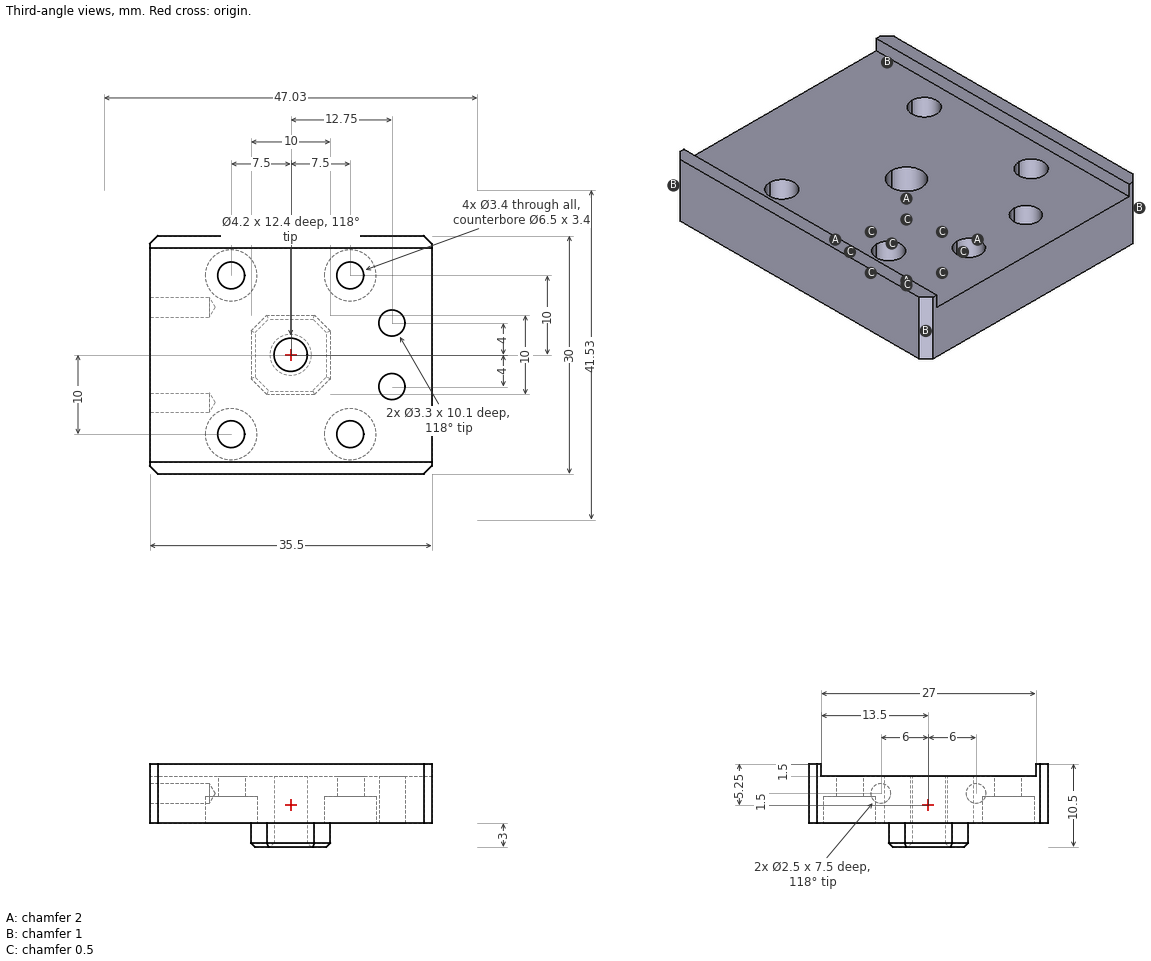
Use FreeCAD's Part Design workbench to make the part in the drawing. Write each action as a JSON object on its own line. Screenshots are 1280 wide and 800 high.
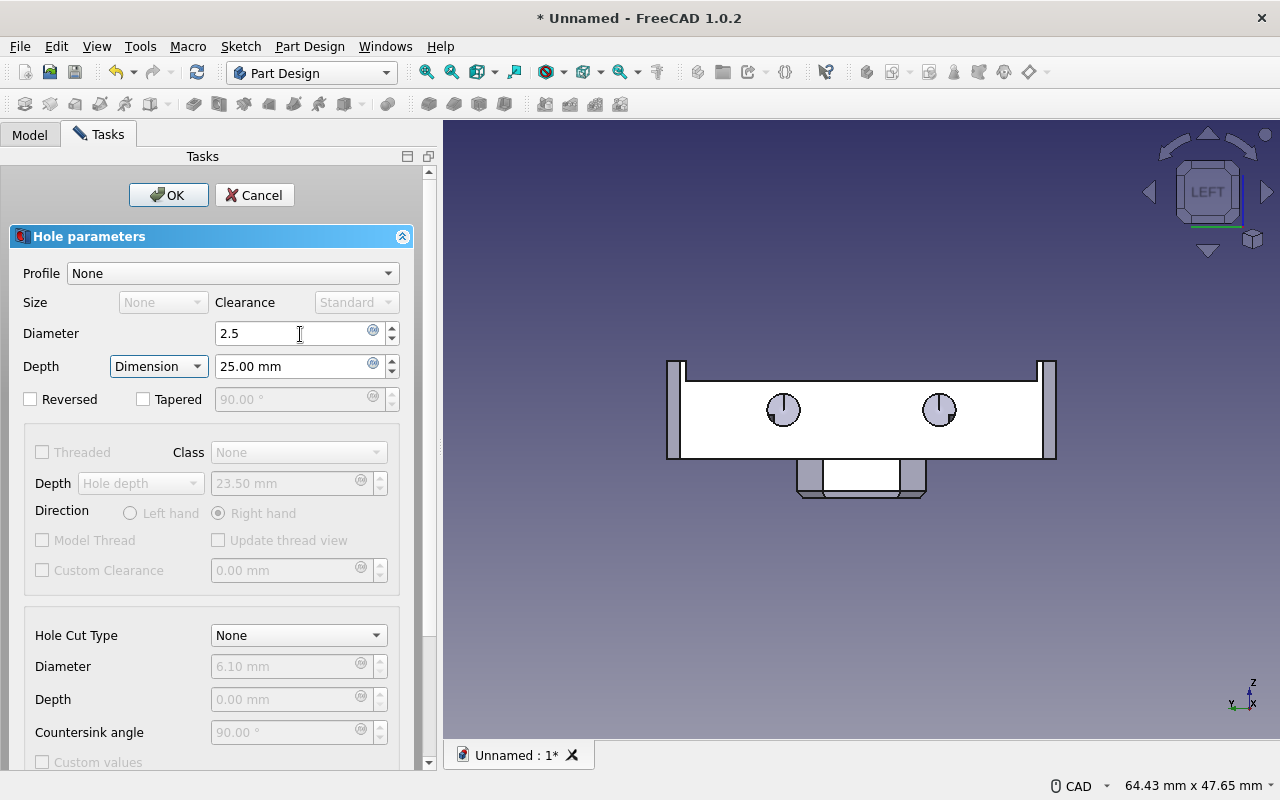
{"action": "triple_click", "coordinate": [300, 366]}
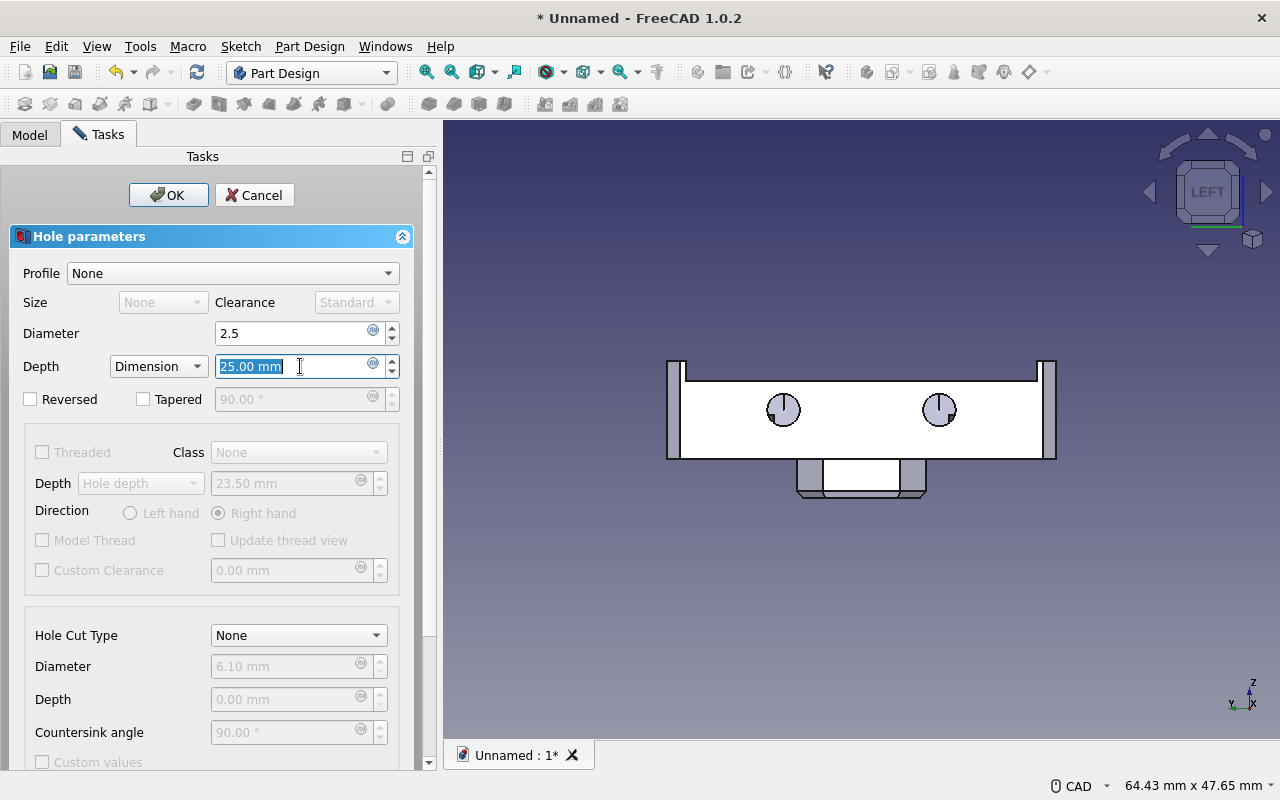
{"action": "type", "text": "7.5"}
{"action": "key", "text": "Tab"}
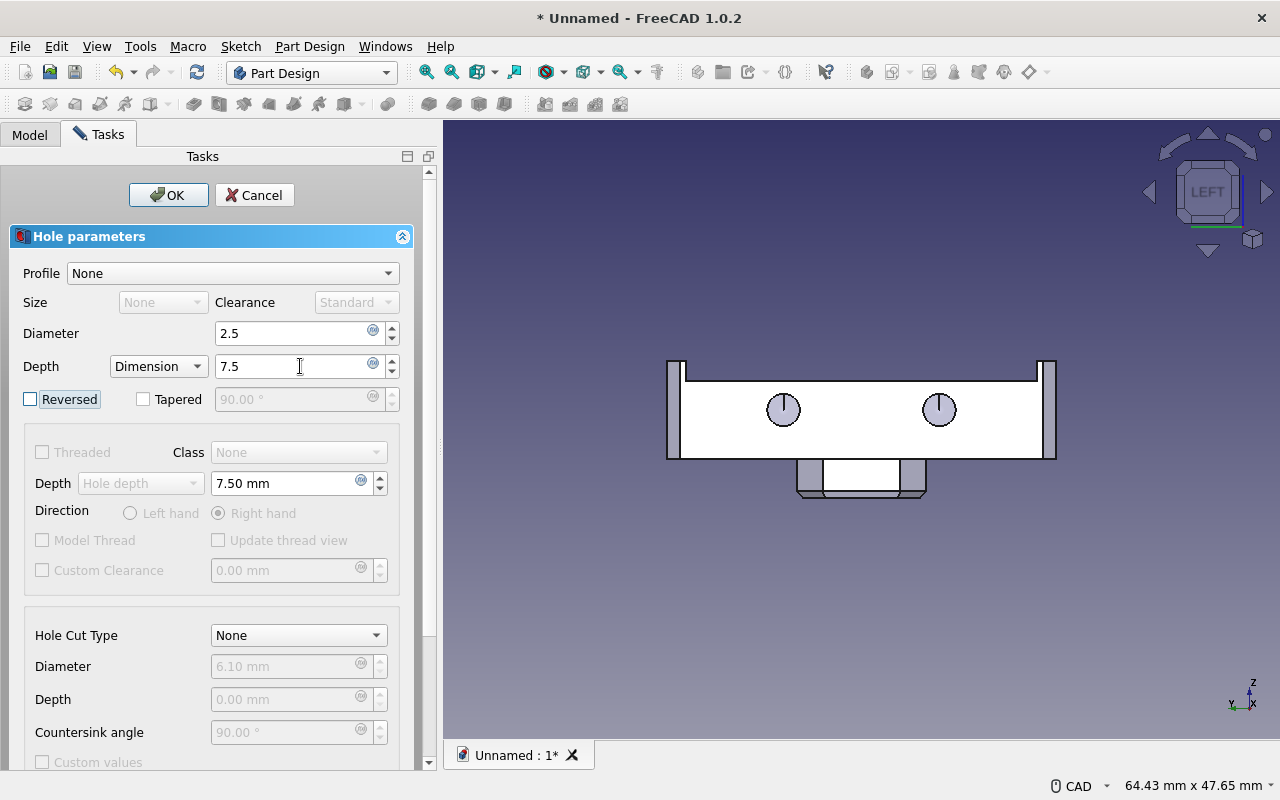
{"action": "left_click", "coordinate": [169, 195]}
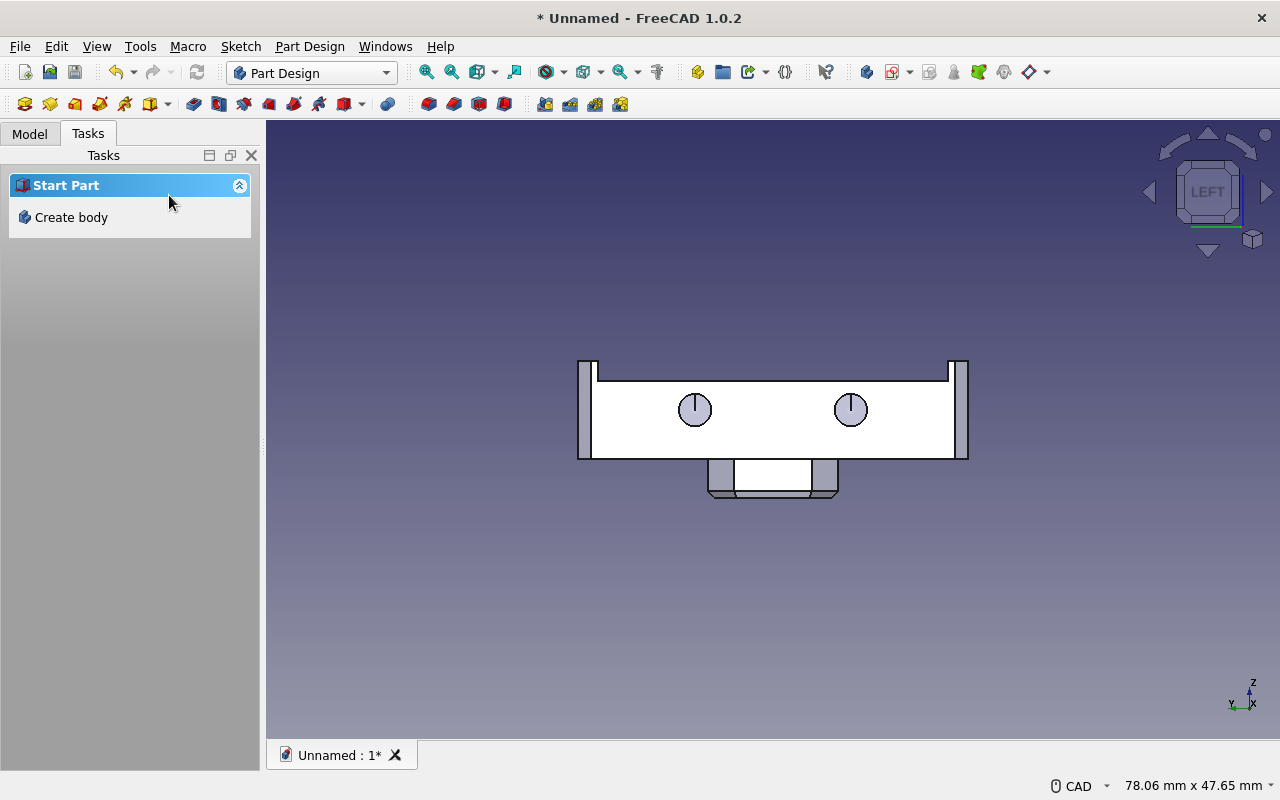
{"action": "key", "text": "0"}